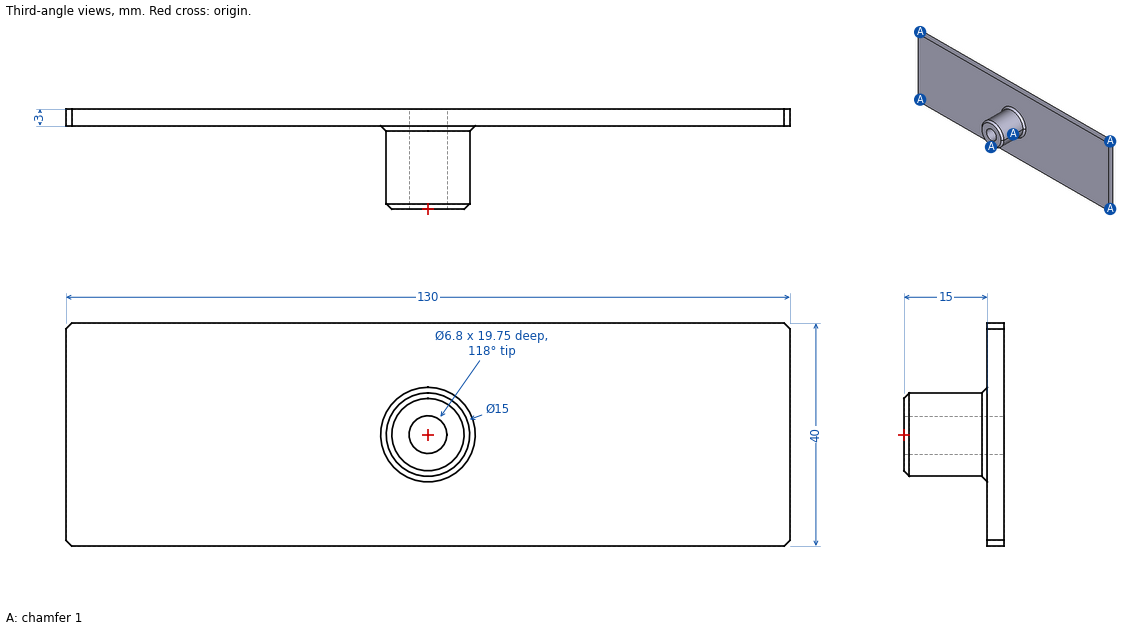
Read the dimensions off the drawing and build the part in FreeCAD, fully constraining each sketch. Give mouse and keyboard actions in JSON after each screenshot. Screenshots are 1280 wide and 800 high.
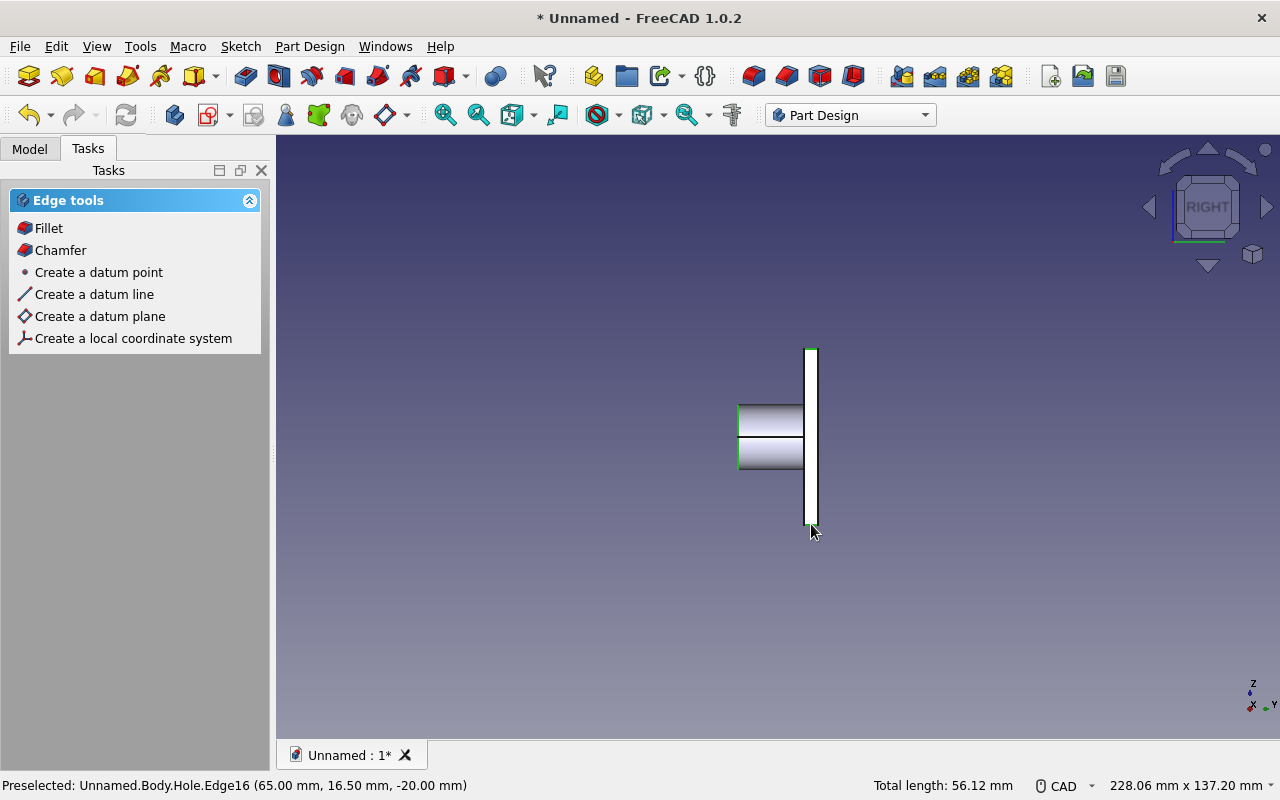
{"action": "key", "text": "5"}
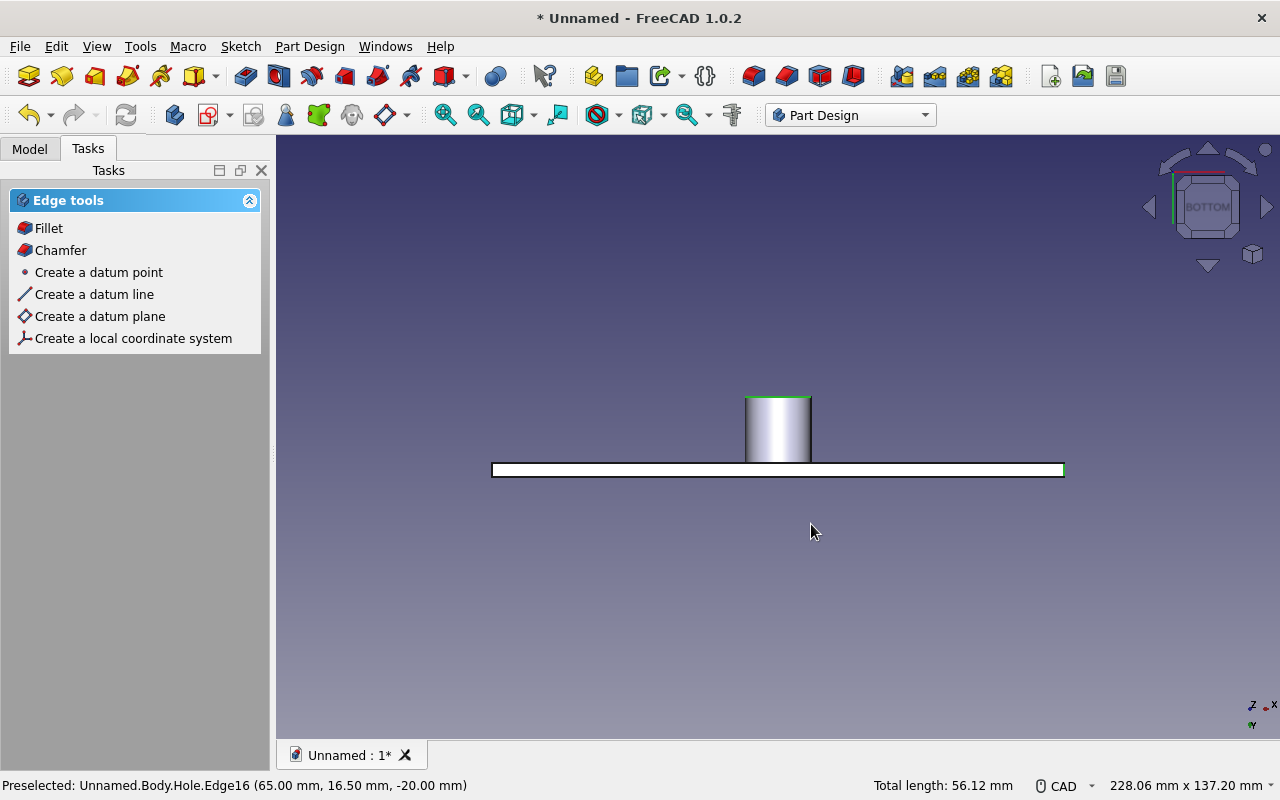
{"action": "left_click", "coordinate": [492, 469], "text": "ctrl"}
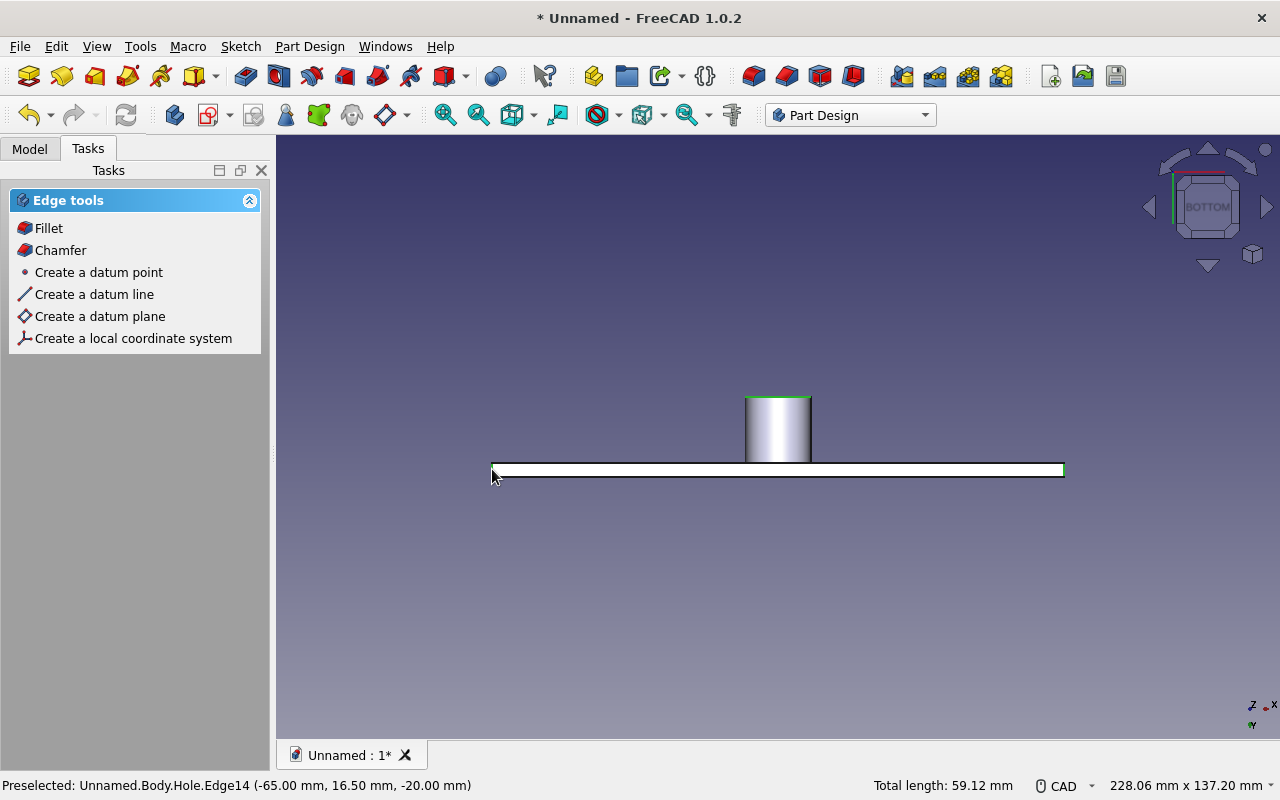
{"action": "key", "text": "4"}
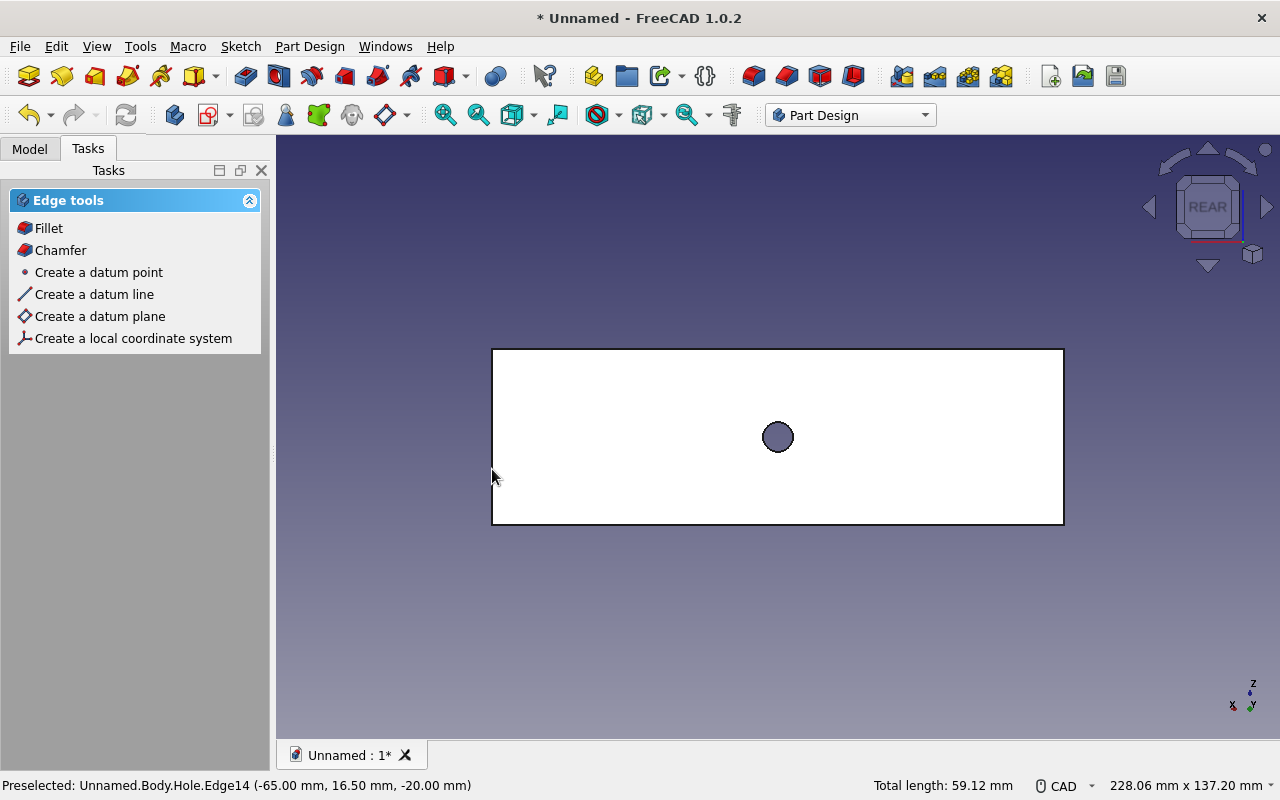
{"action": "key", "text": "6"}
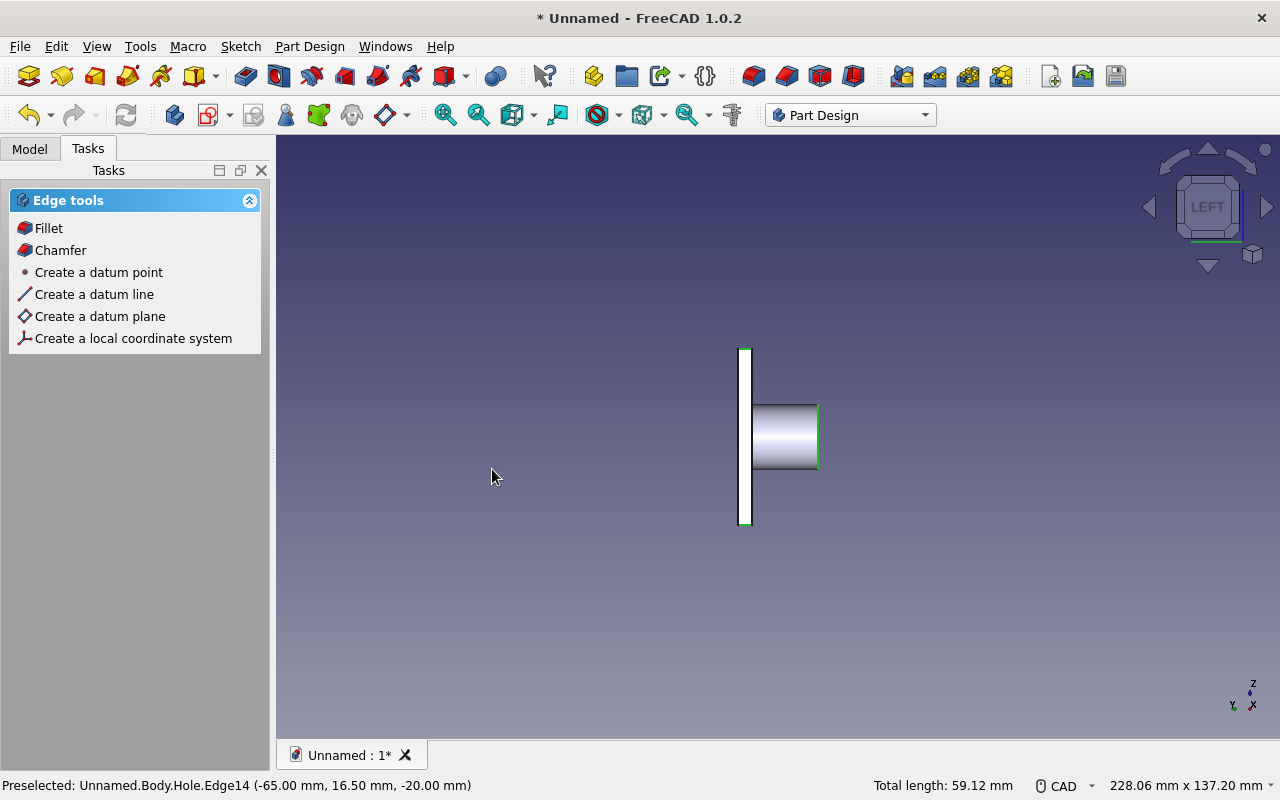
{"action": "left_click", "coordinate": [446, 116]}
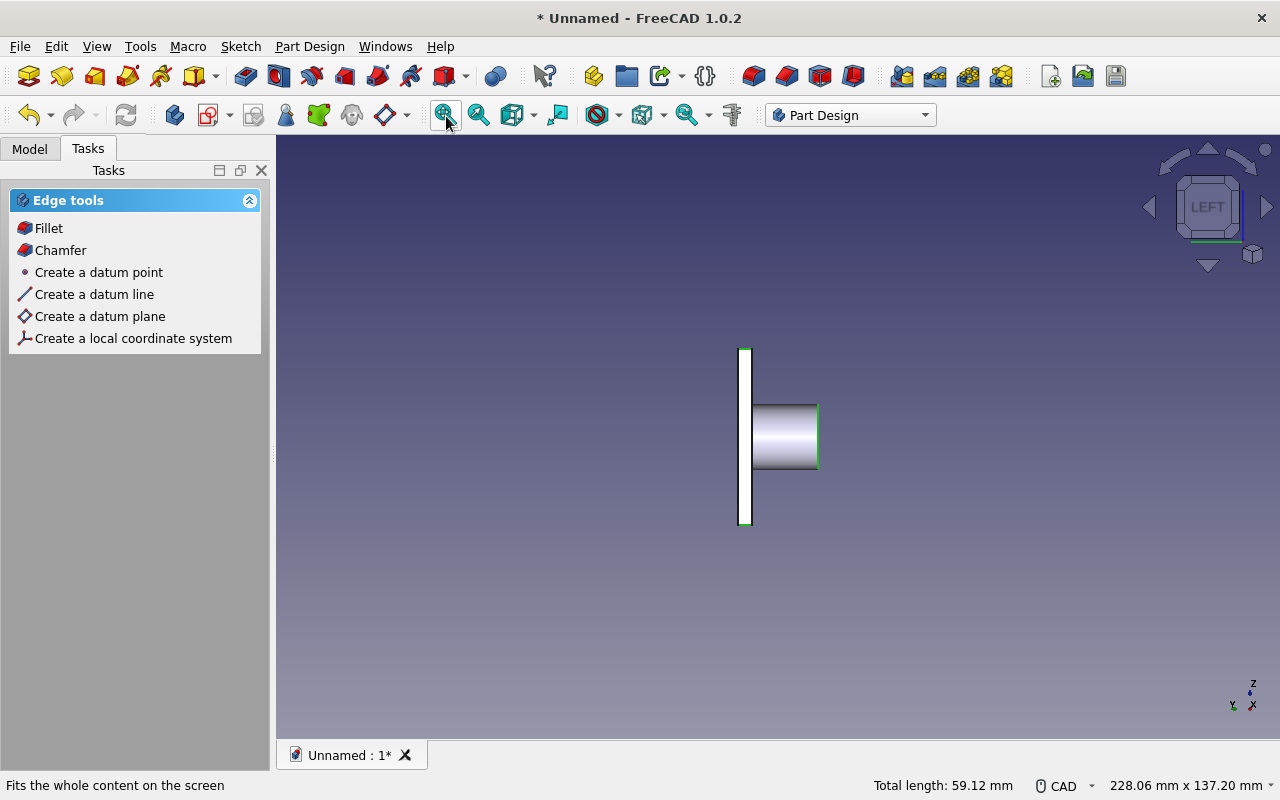
{"action": "key", "text": "v 3"}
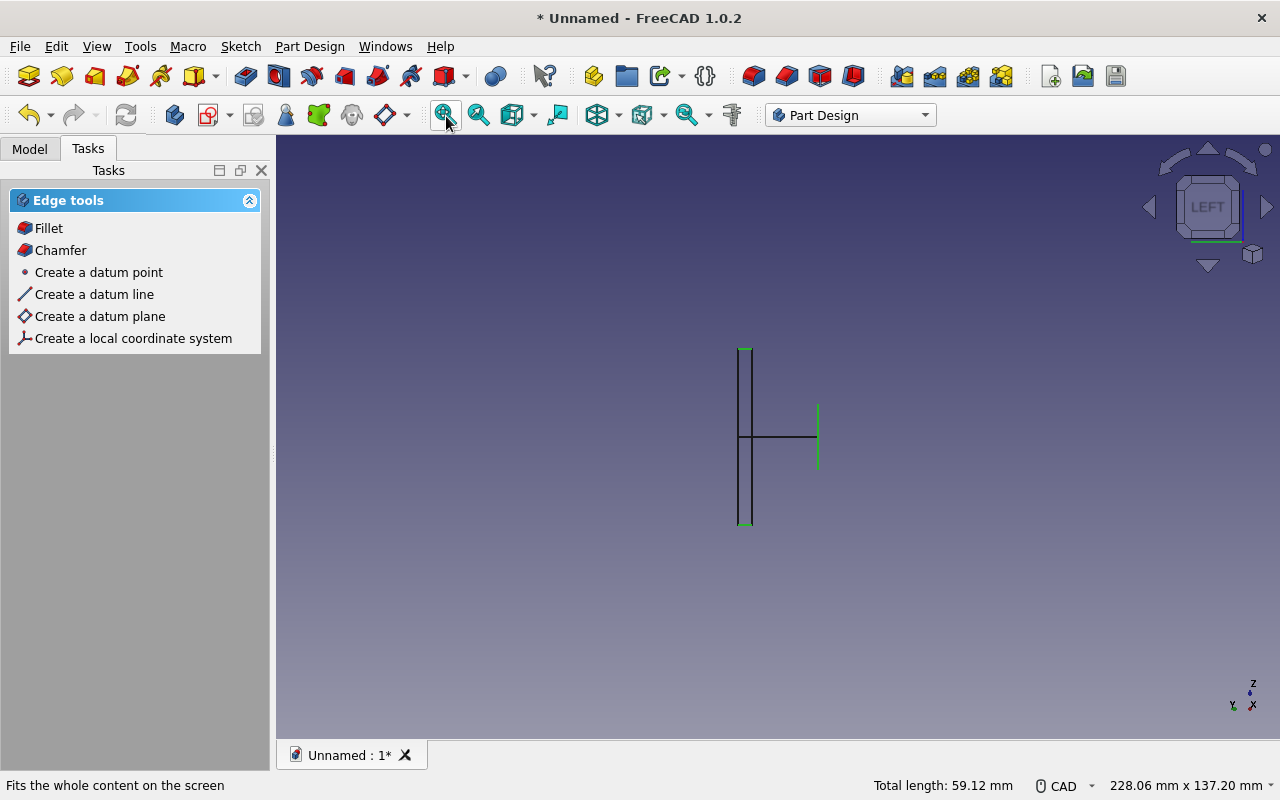
{"action": "key", "text": "0"}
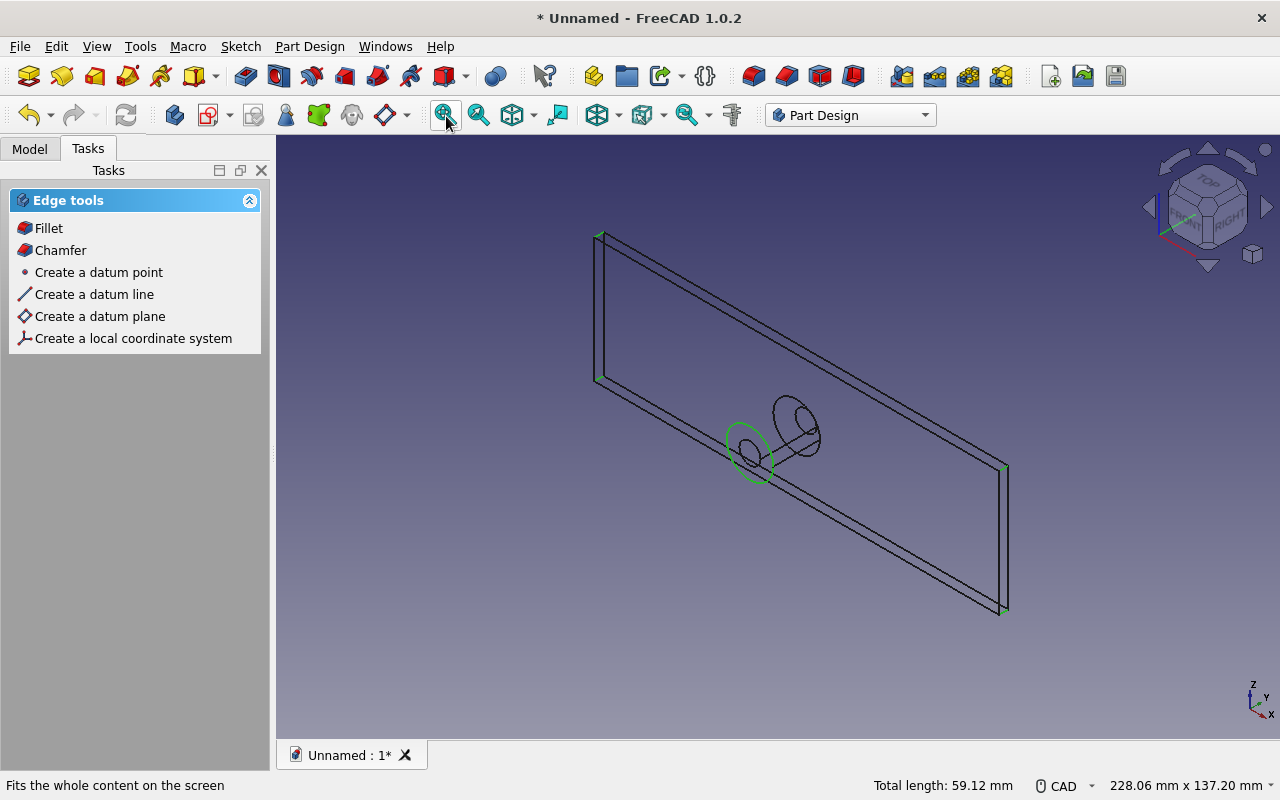
{"action": "left_click", "coordinate": [773, 412], "text": "ctrl"}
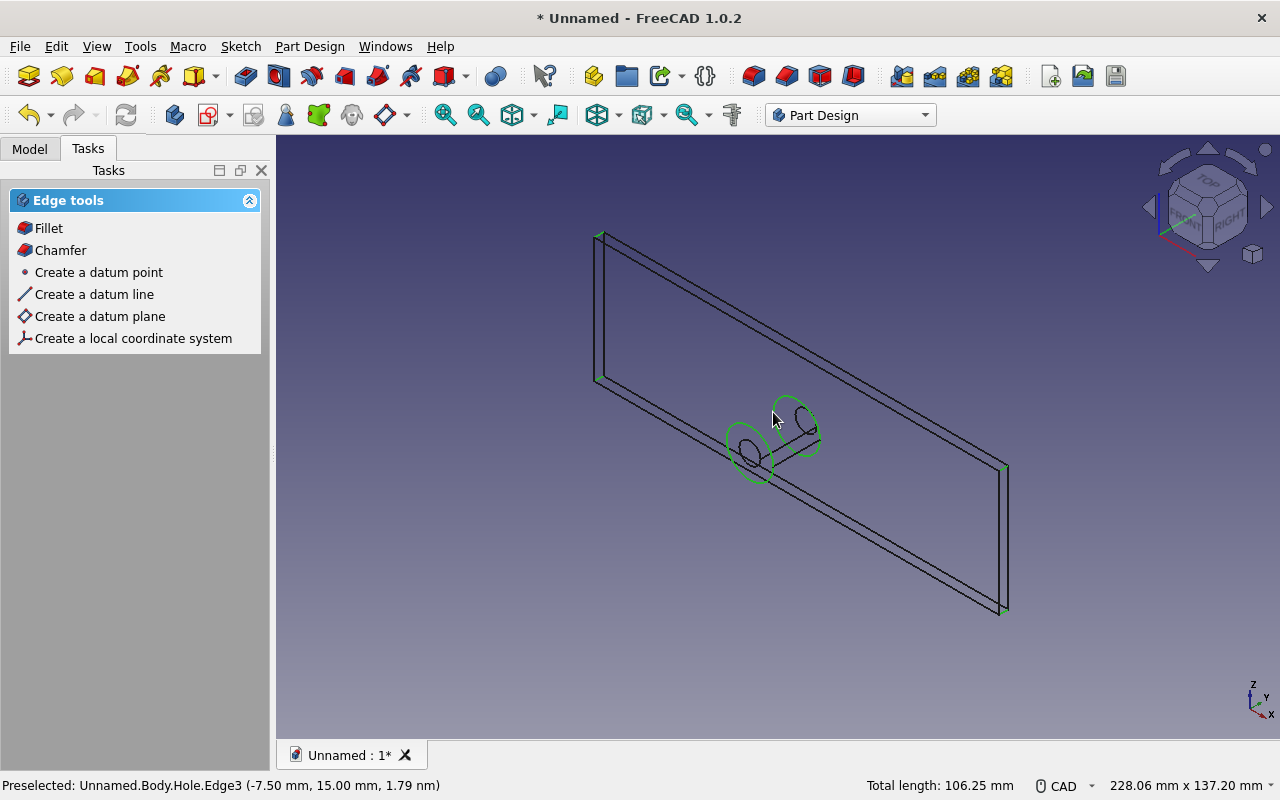
{"action": "key", "text": "v 1"}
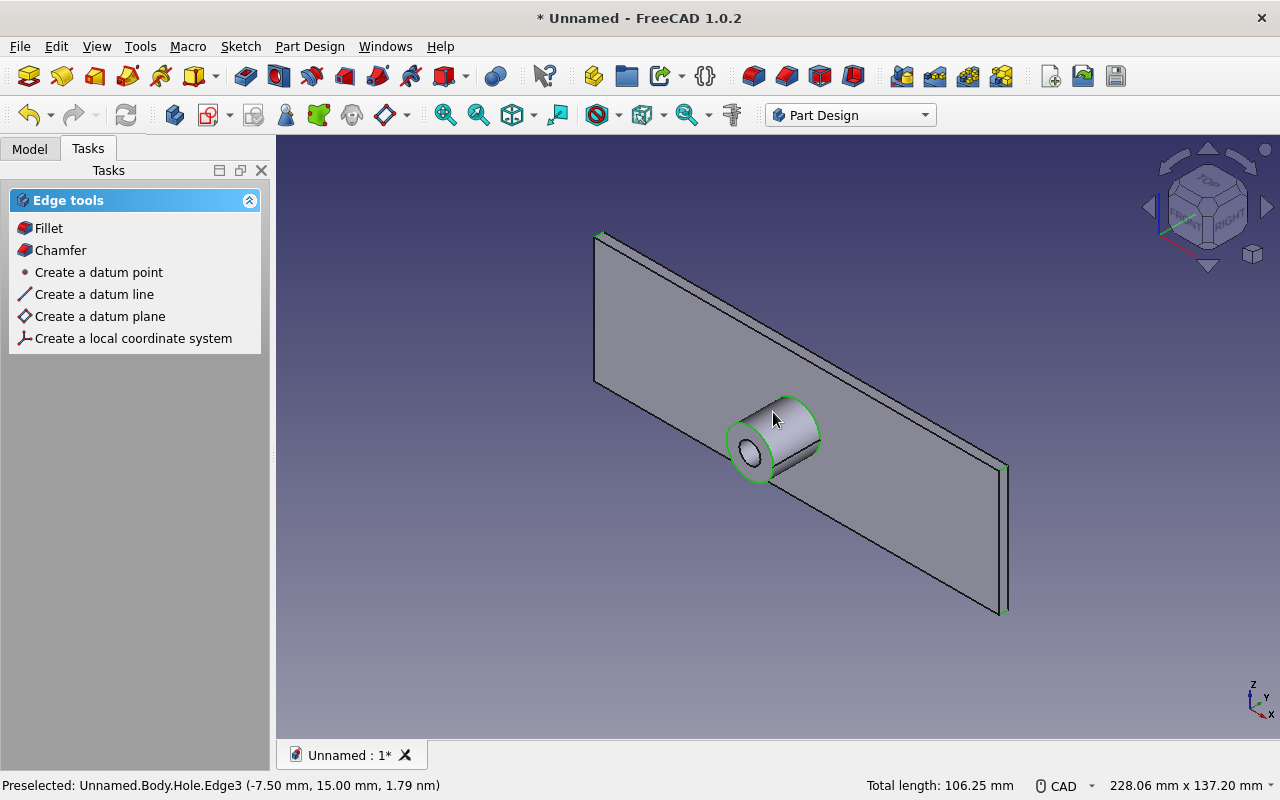
{"action": "left_click", "coordinate": [787, 76]}